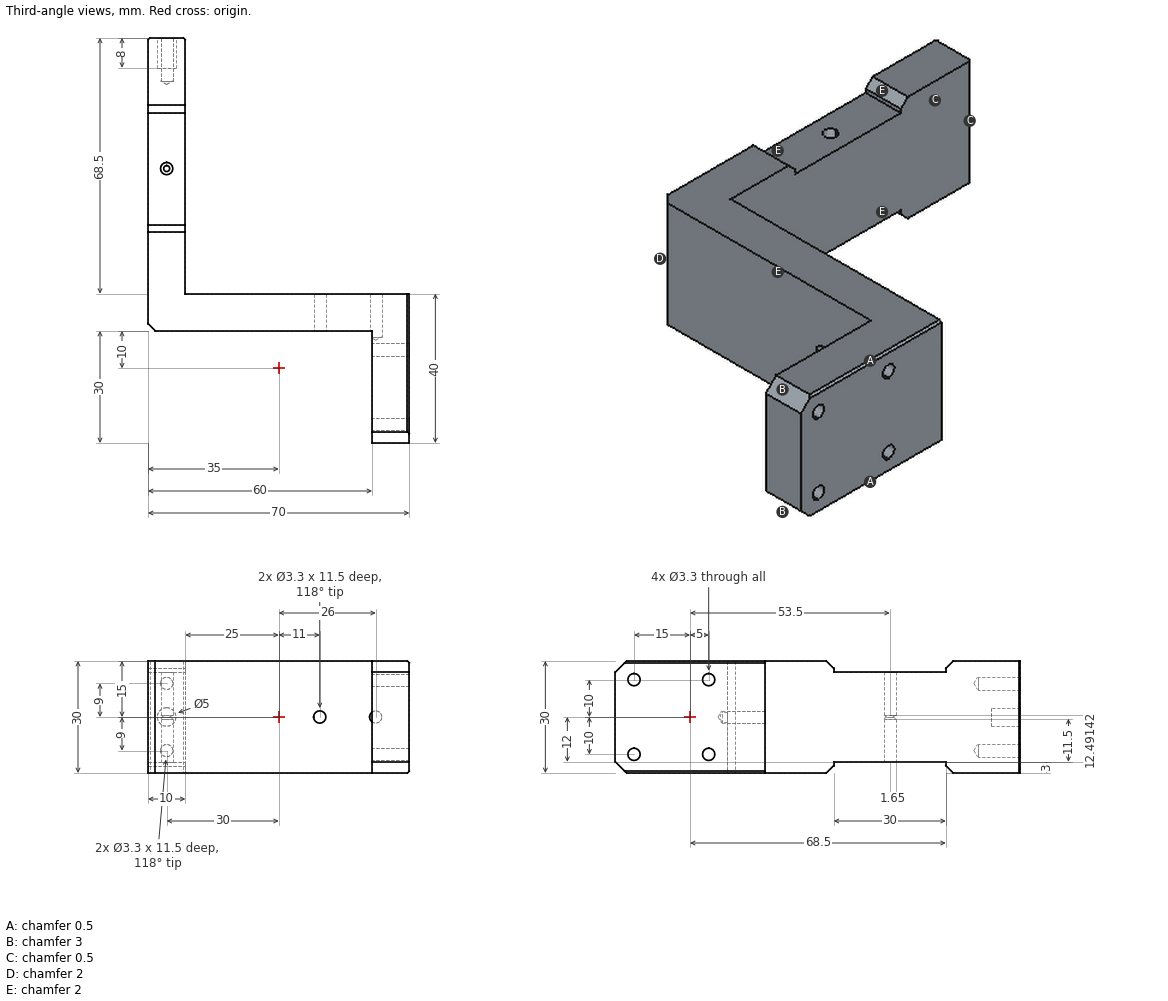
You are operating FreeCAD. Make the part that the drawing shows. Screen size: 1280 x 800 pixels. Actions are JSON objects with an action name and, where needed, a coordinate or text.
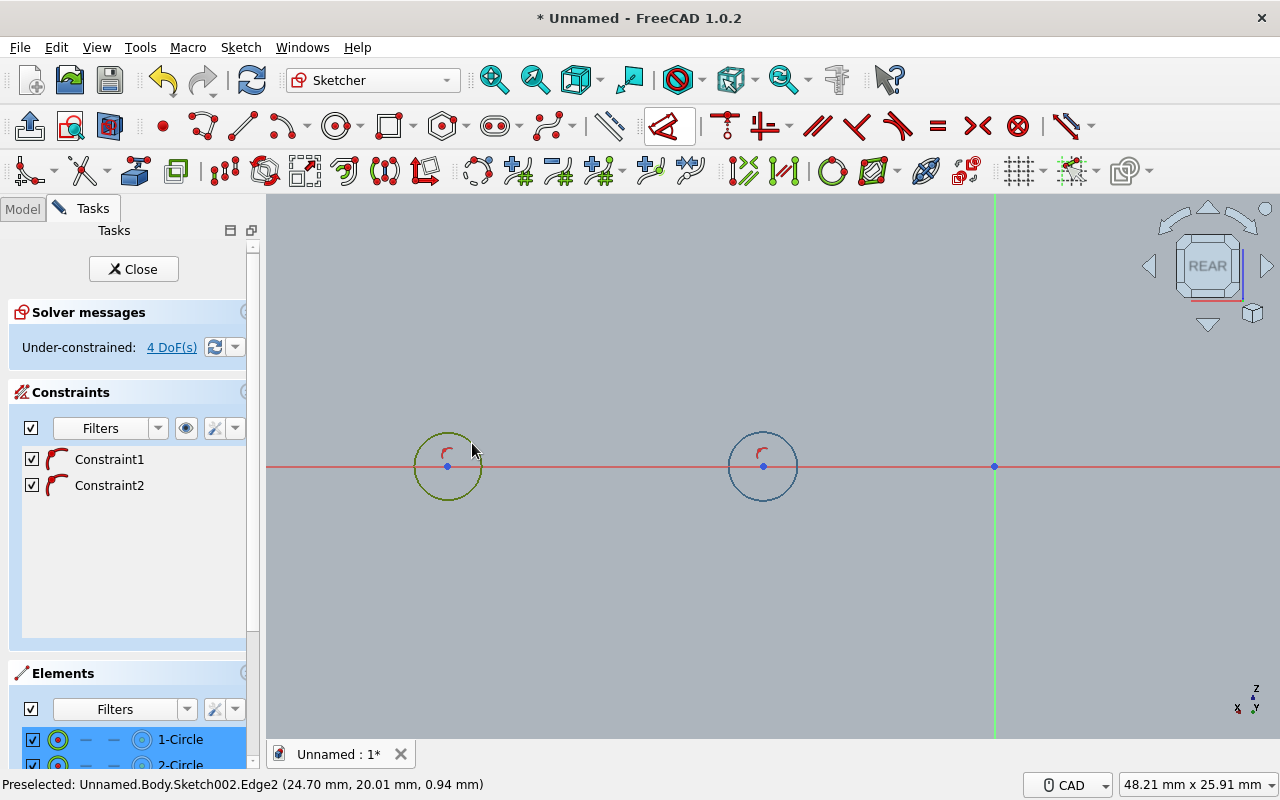
{"action": "left_click", "coordinate": [938, 126]}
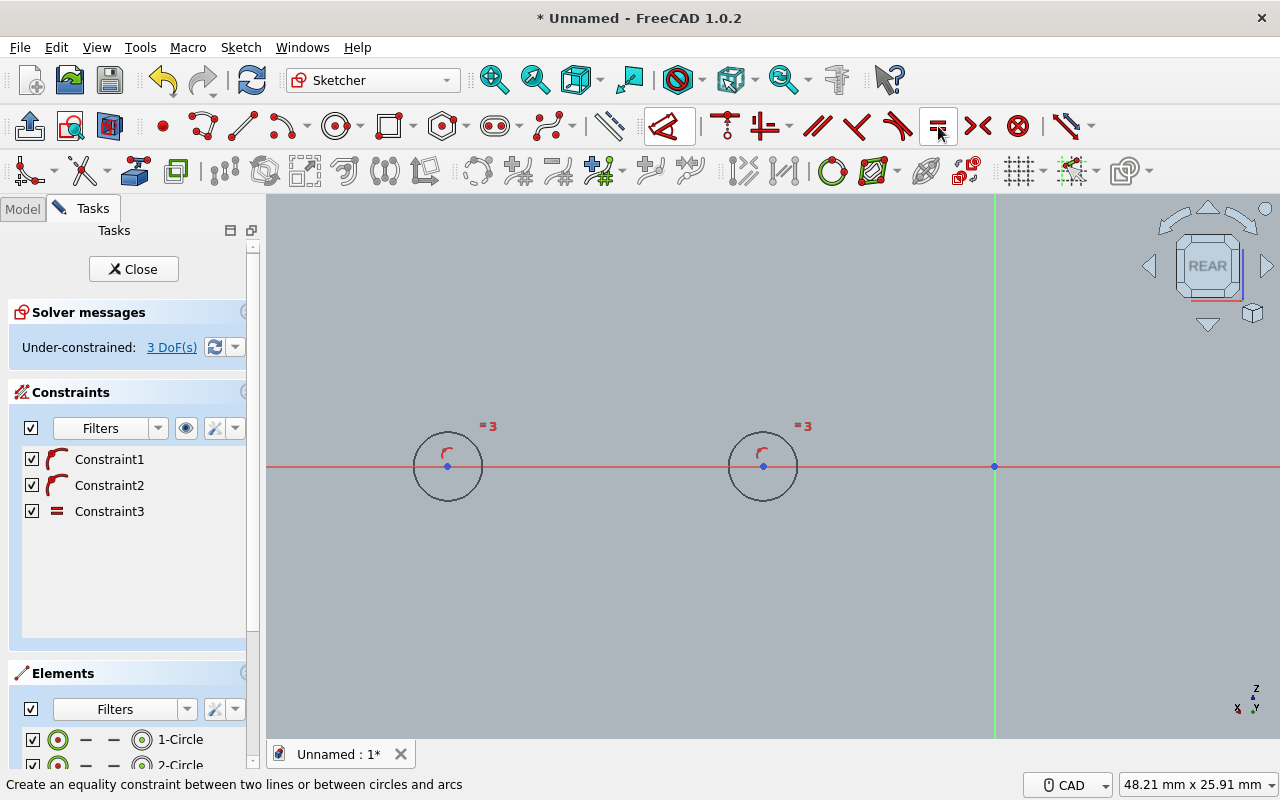
{"action": "left_click", "coordinate": [787, 442]}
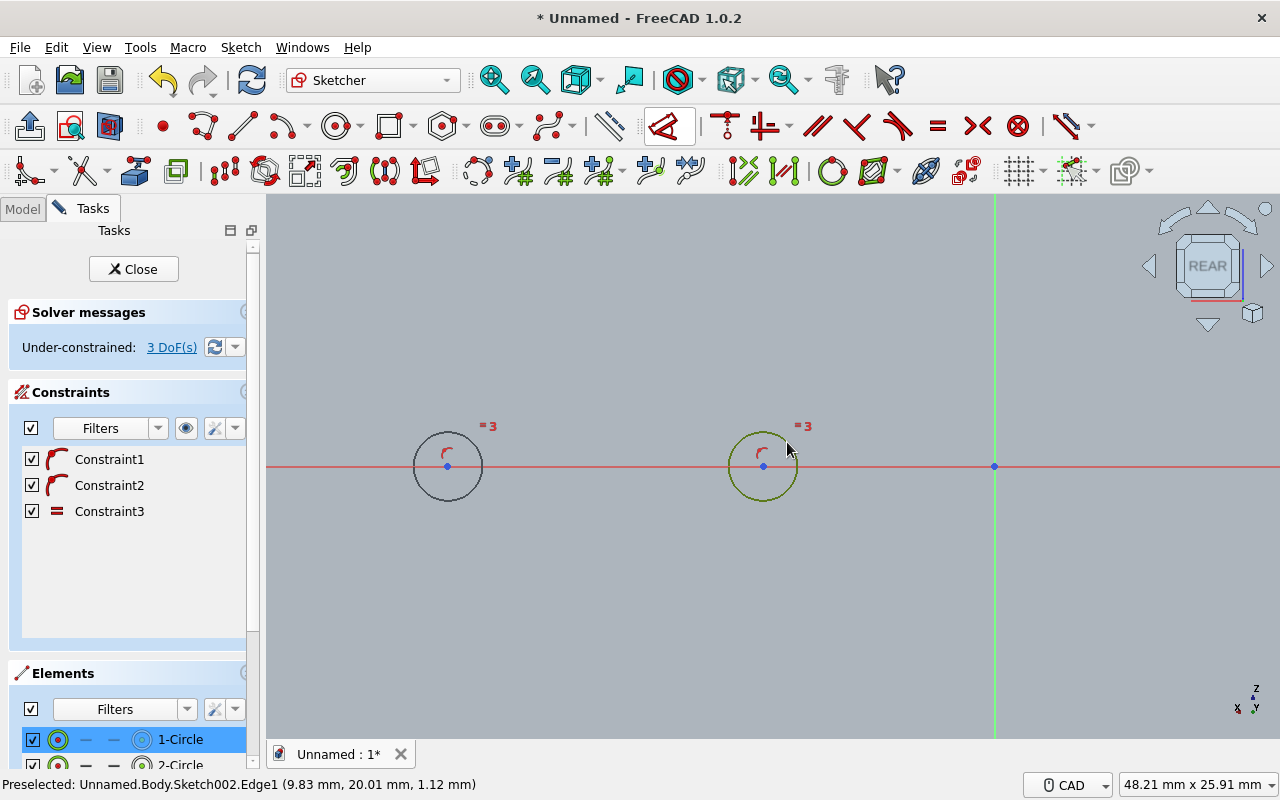
{"action": "key", "text": "k o"}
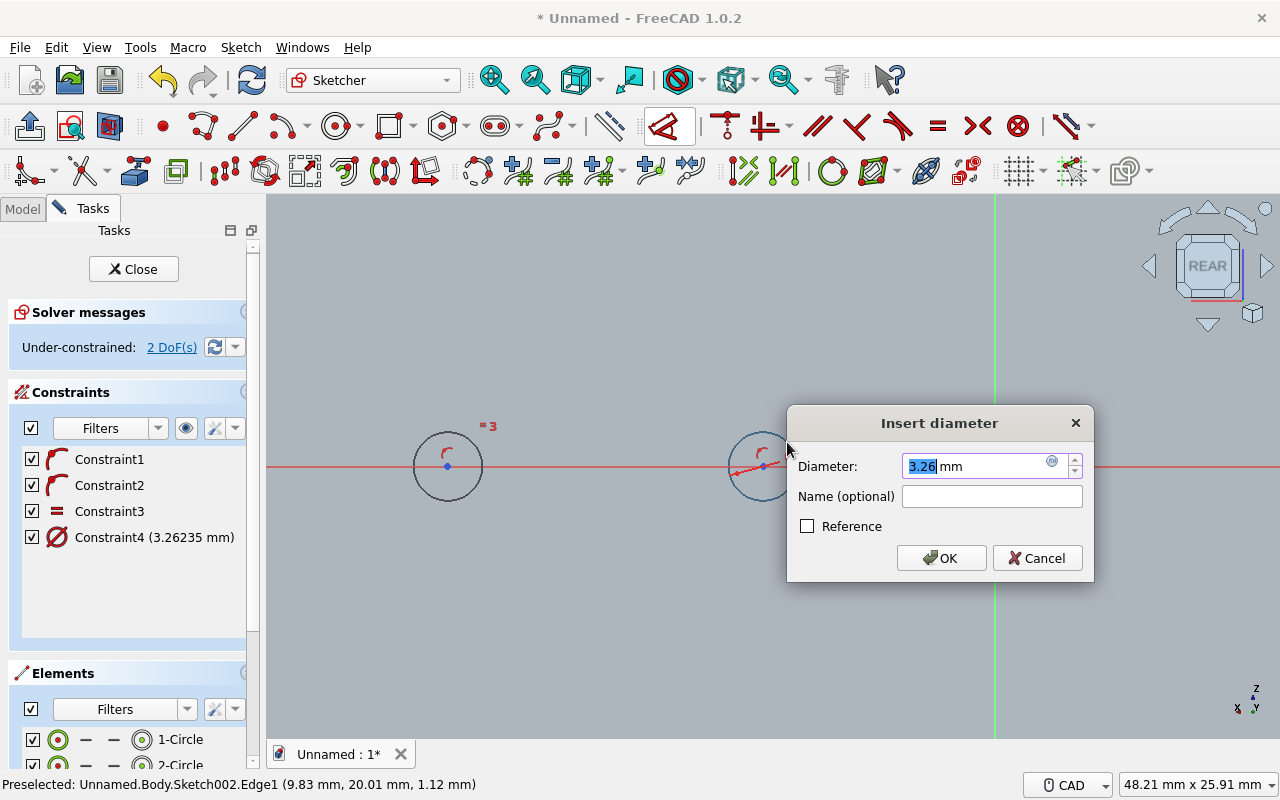
{"action": "type", "text": "3.3"}
{"action": "key", "text": "Return"}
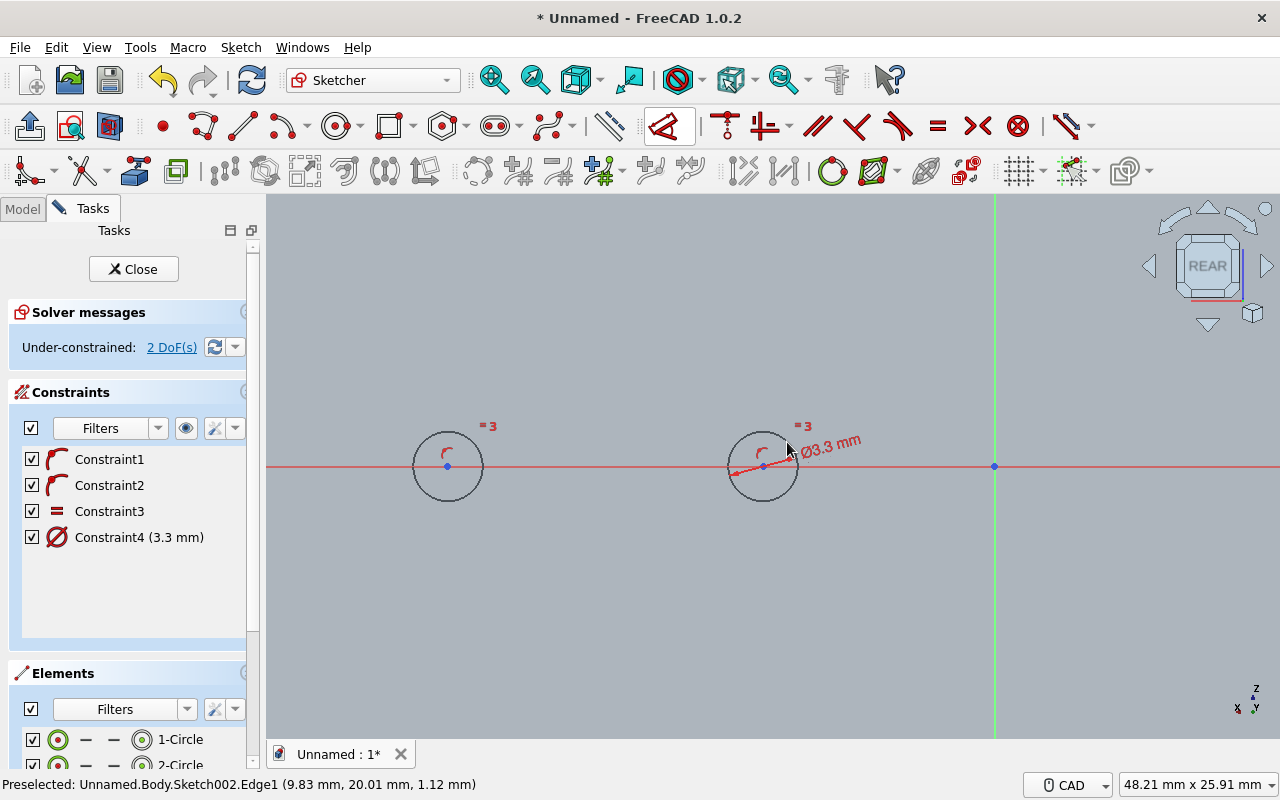
{"action": "left_click", "coordinate": [763, 466]}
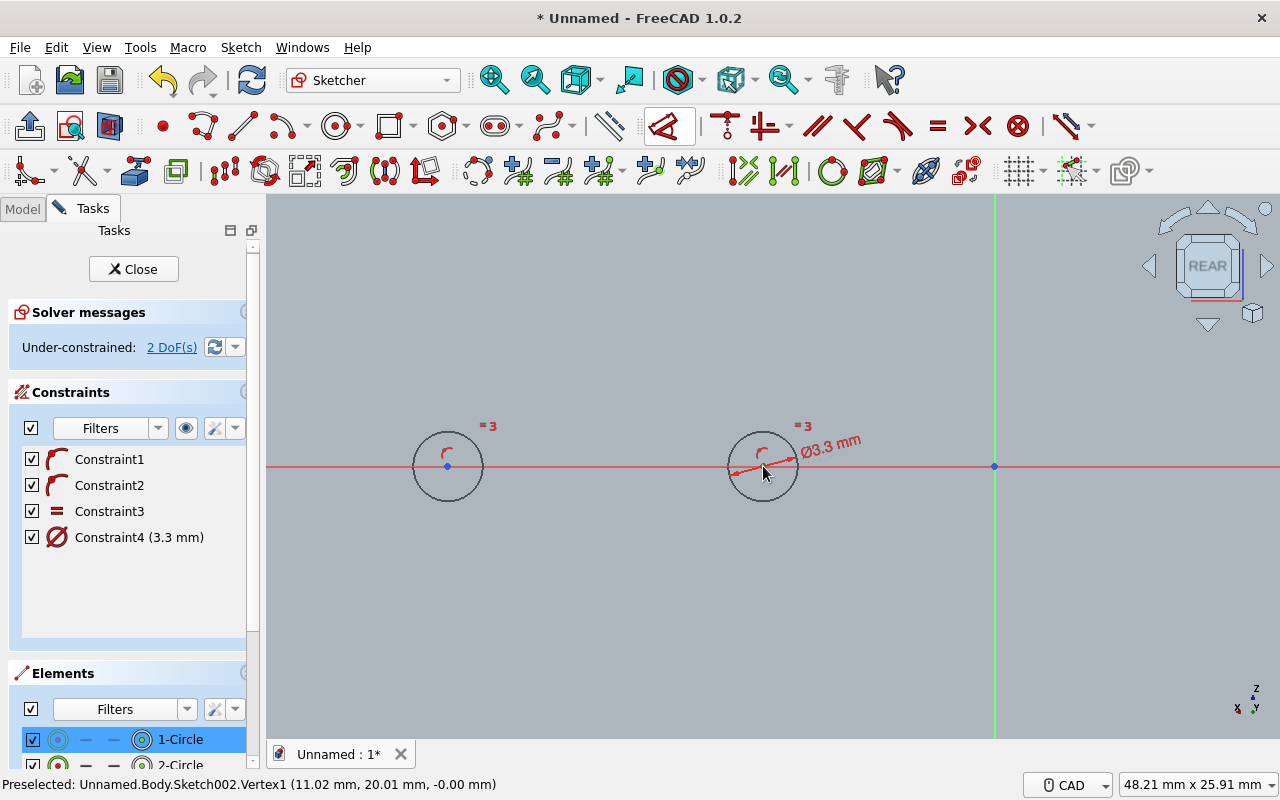
{"action": "key", "text": "l"}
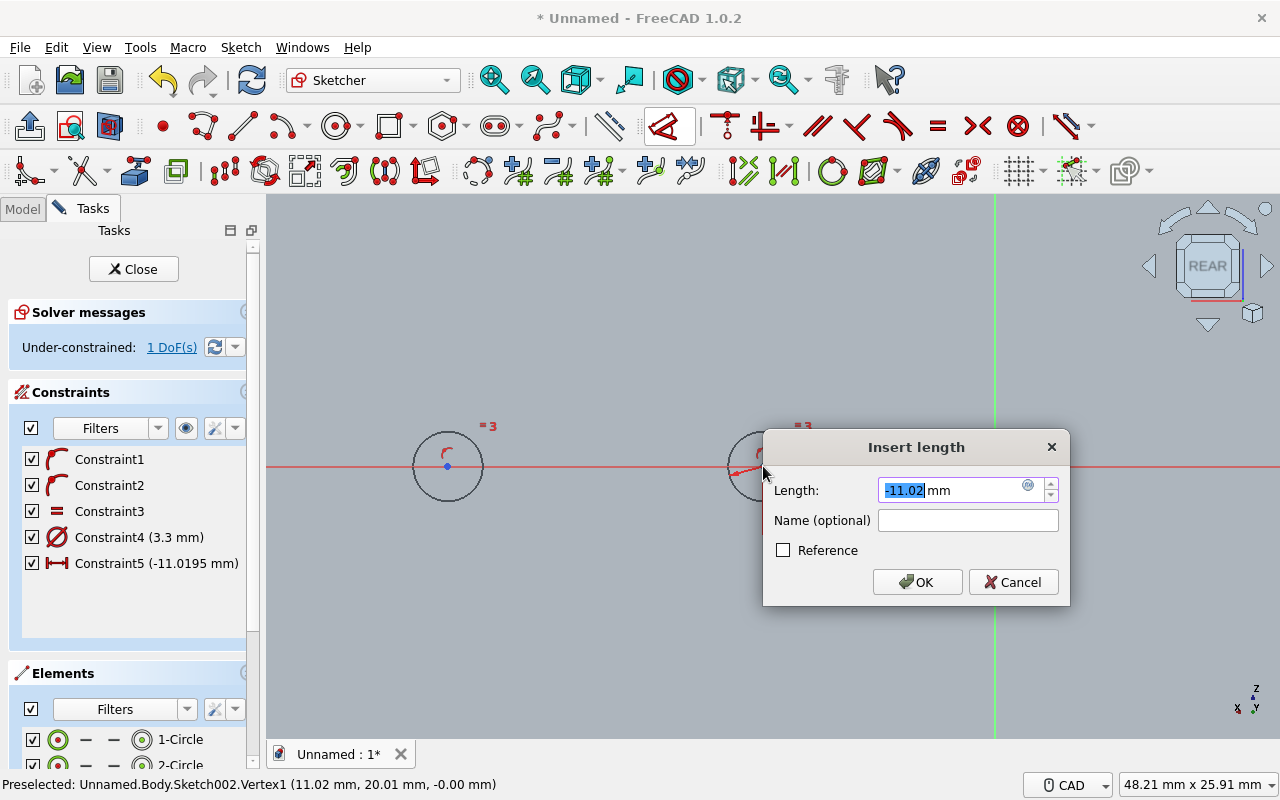
{"action": "type", "text": "-11"}
{"action": "key", "text": "Return"}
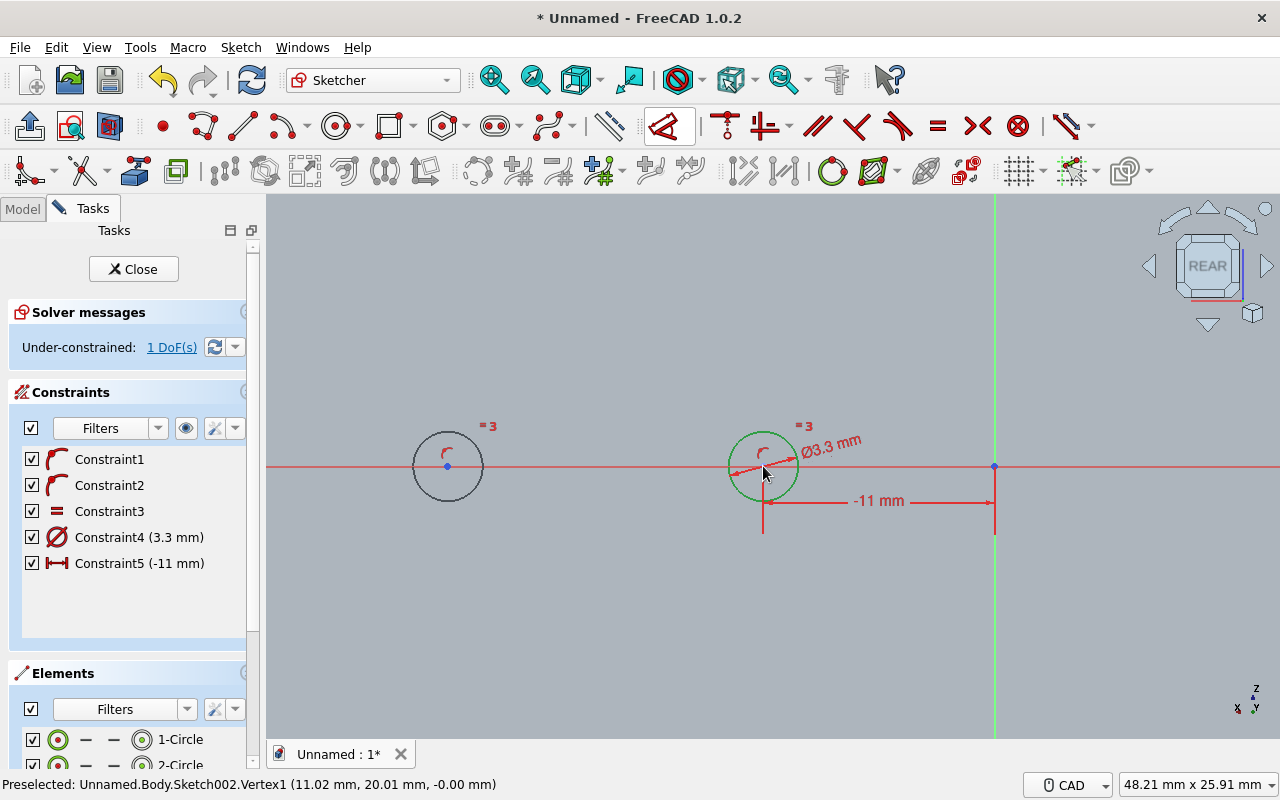
{"action": "left_click", "coordinate": [448, 466]}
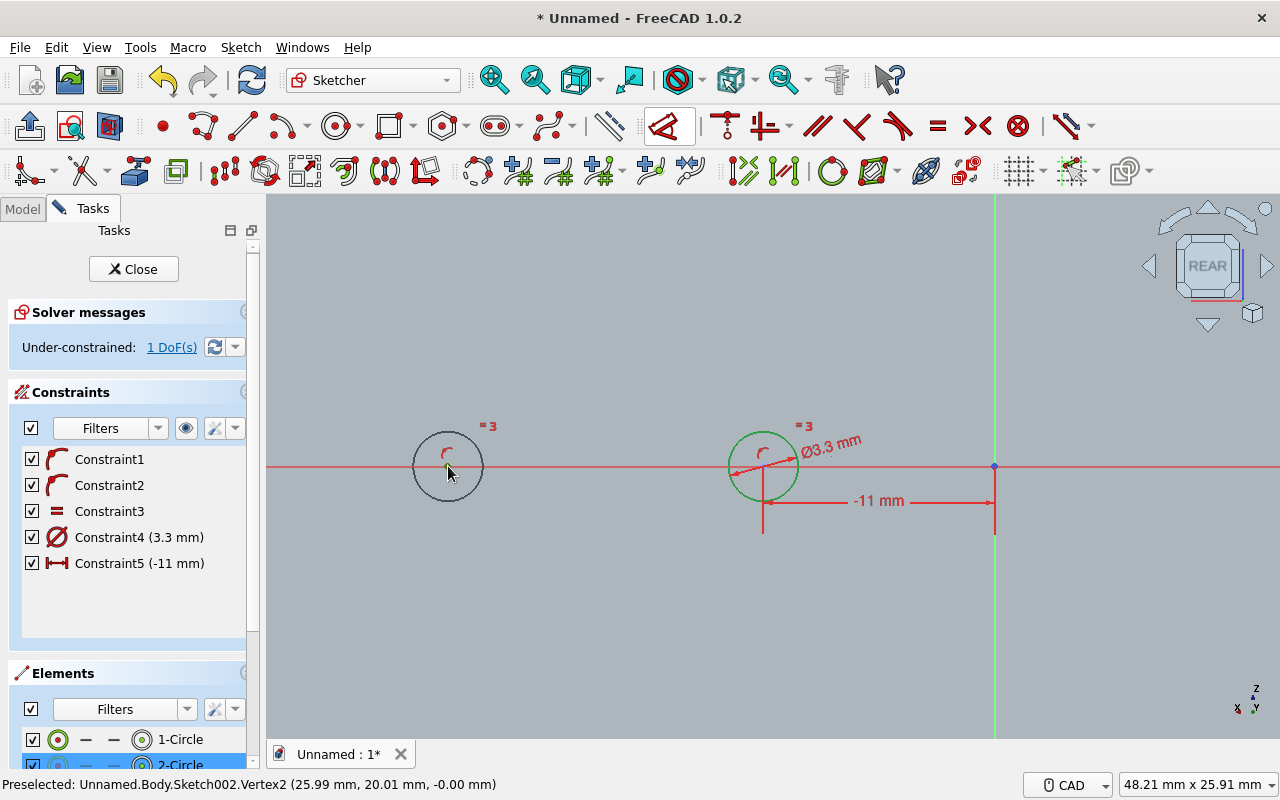
{"action": "key", "text": "l"}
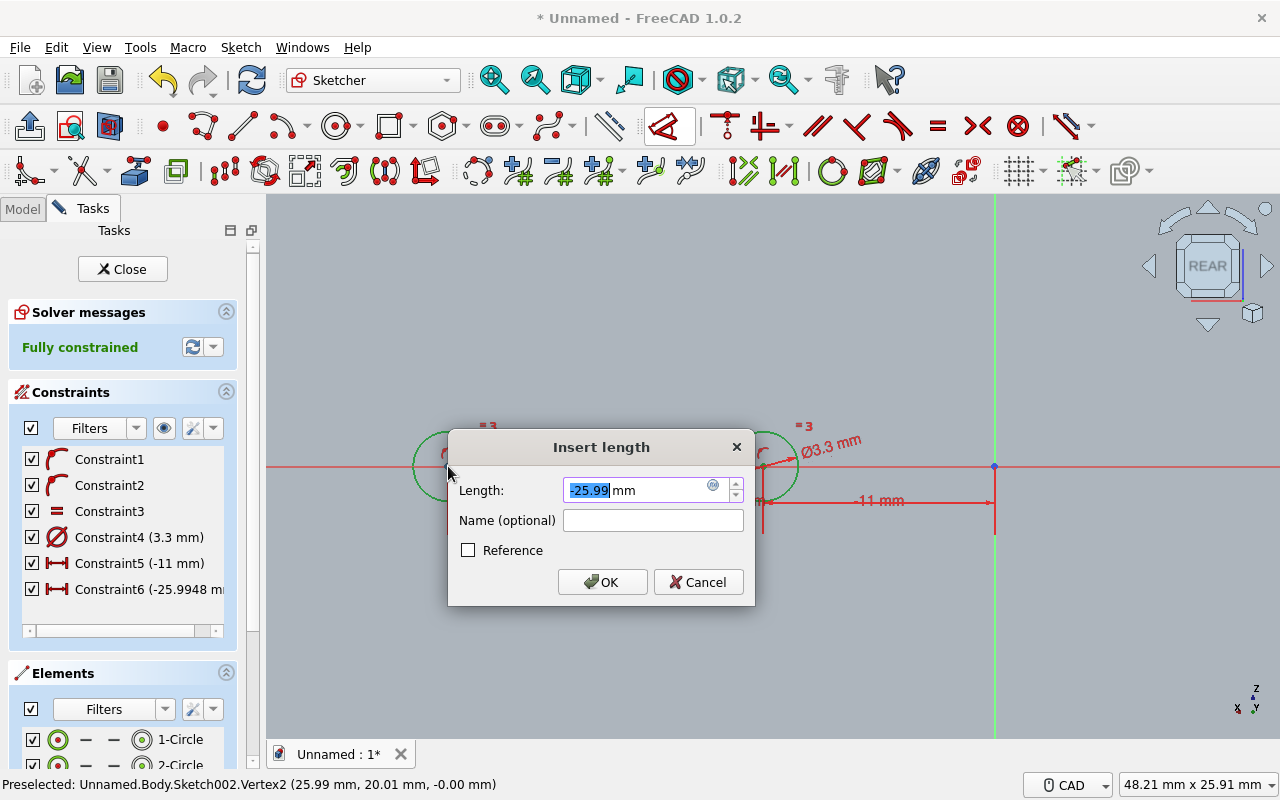
{"action": "type", "text": "-26"}
{"action": "key", "text": "Return"}